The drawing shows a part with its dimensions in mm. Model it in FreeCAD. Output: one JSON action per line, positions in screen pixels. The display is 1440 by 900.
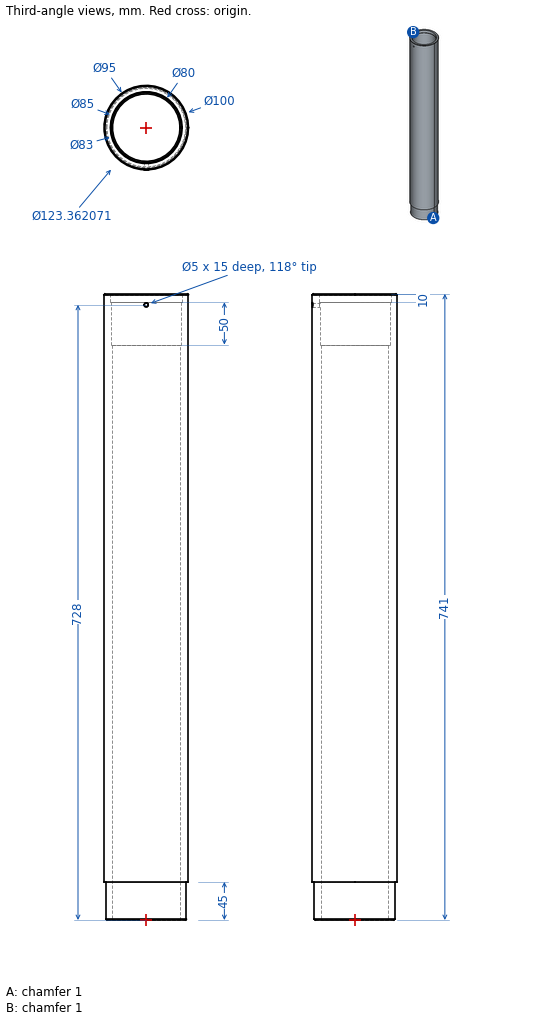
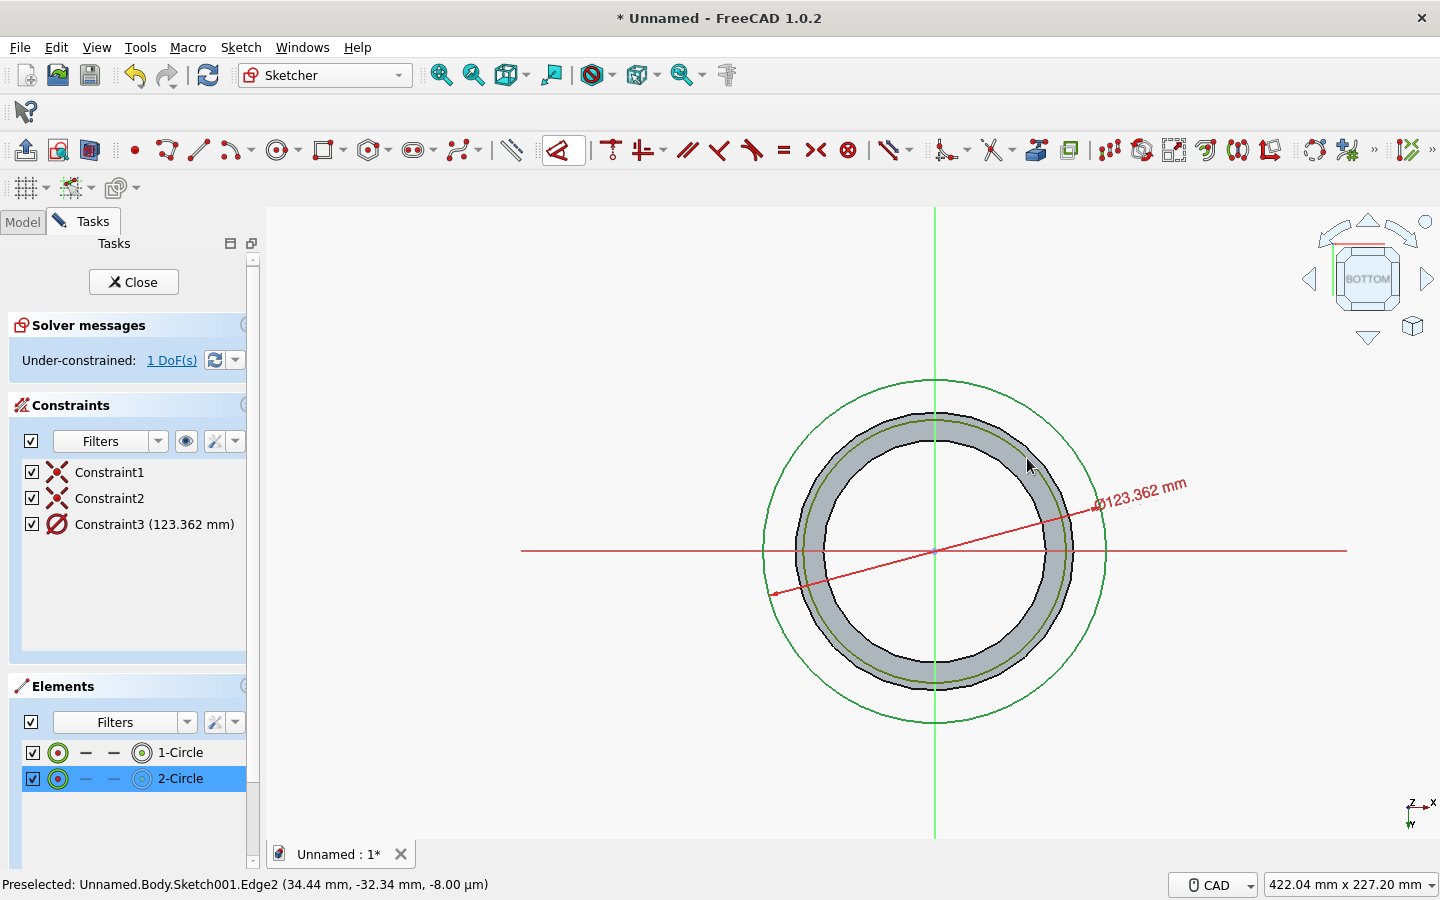
{"action": "left_click", "coordinate": [580, 150]}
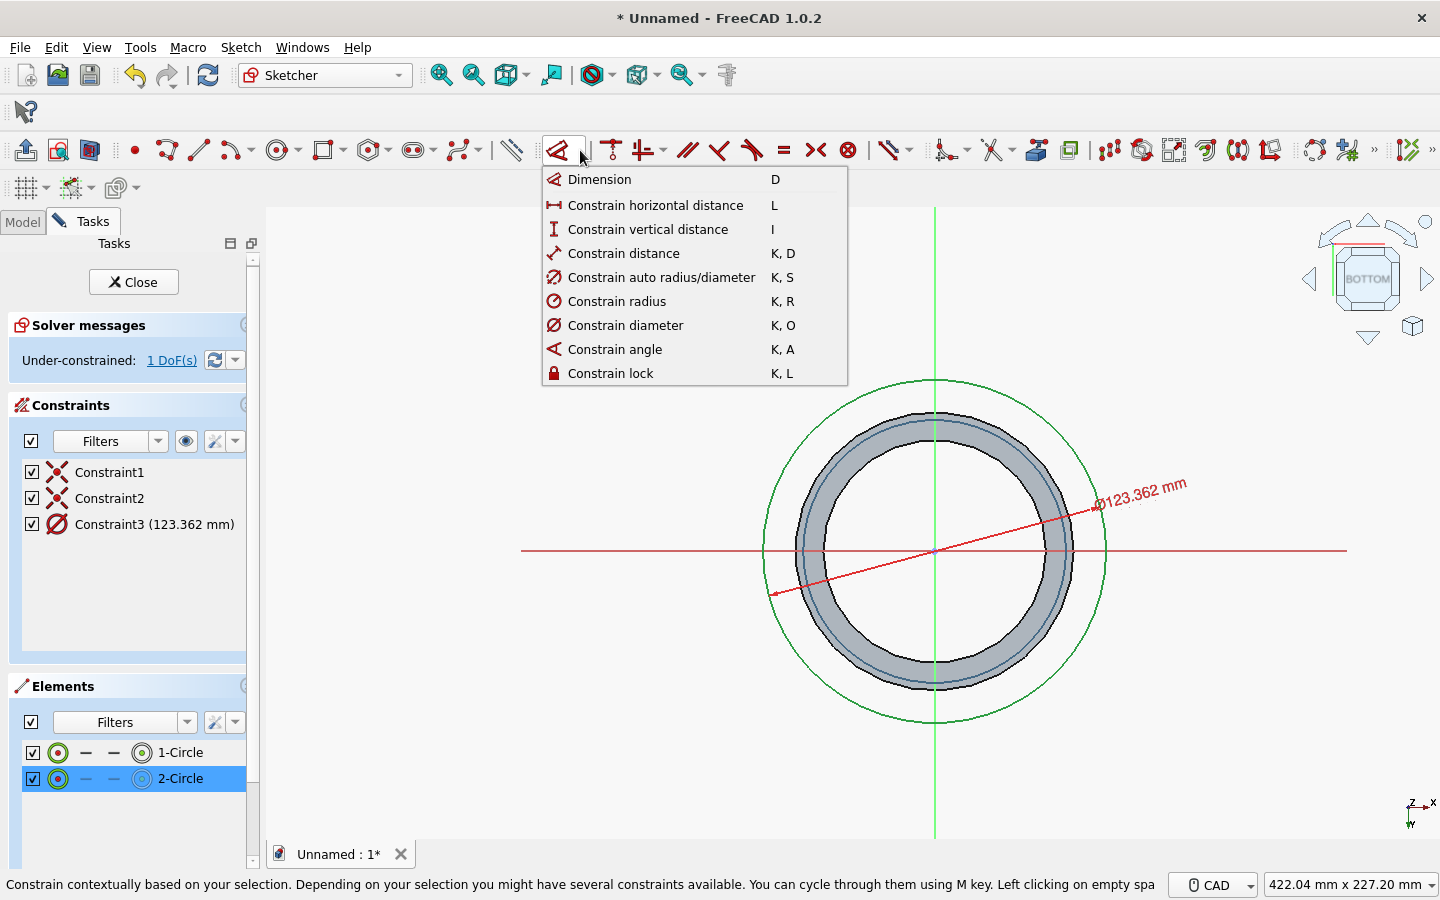
{"action": "left_click", "coordinate": [695, 325]}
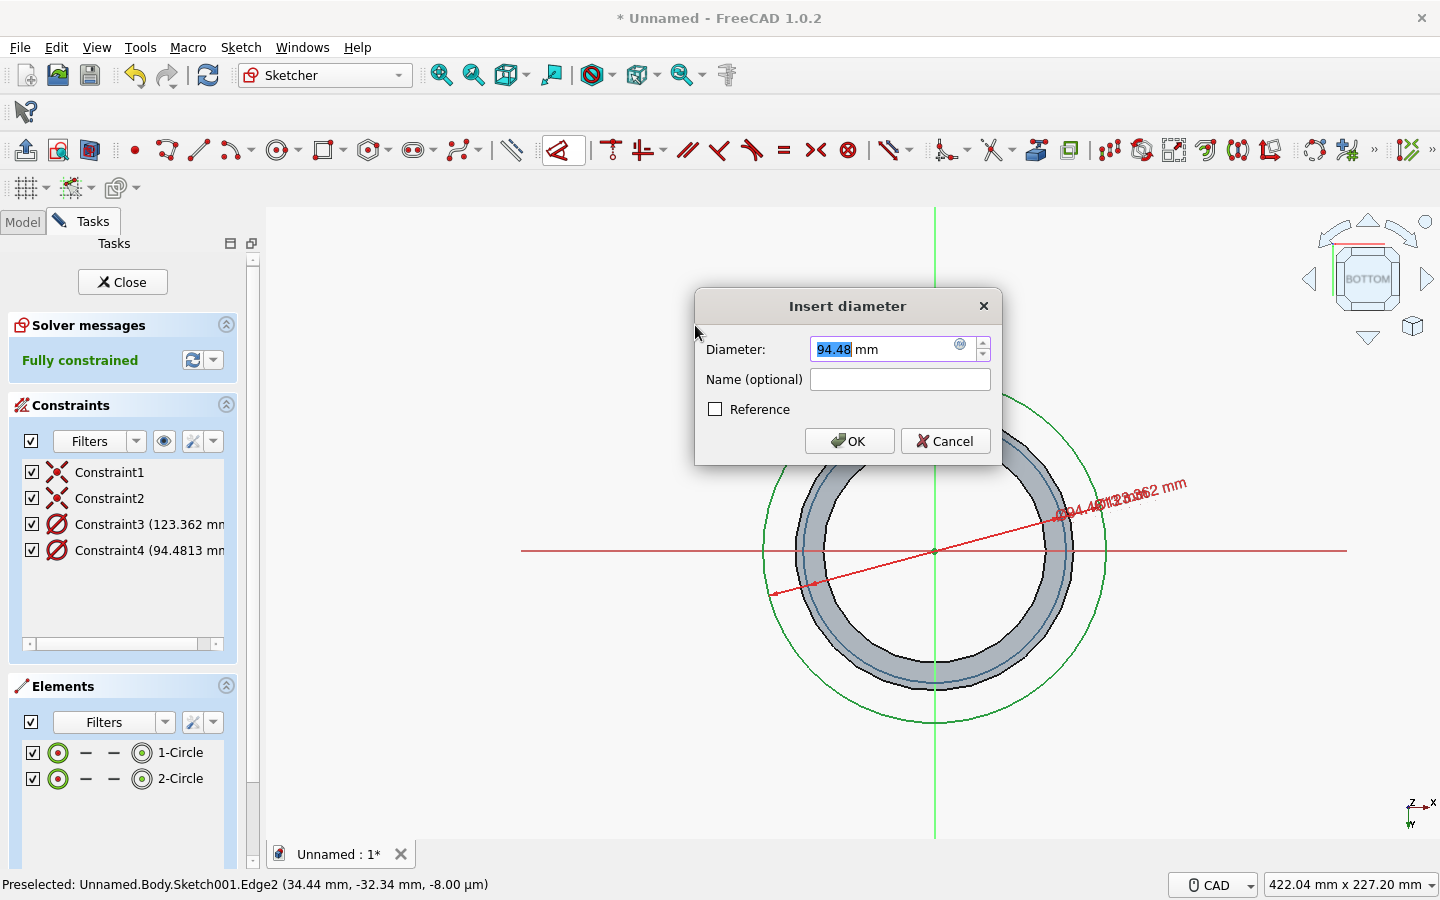
{"action": "type", "text": "95"}
{"action": "key", "text": "Return"}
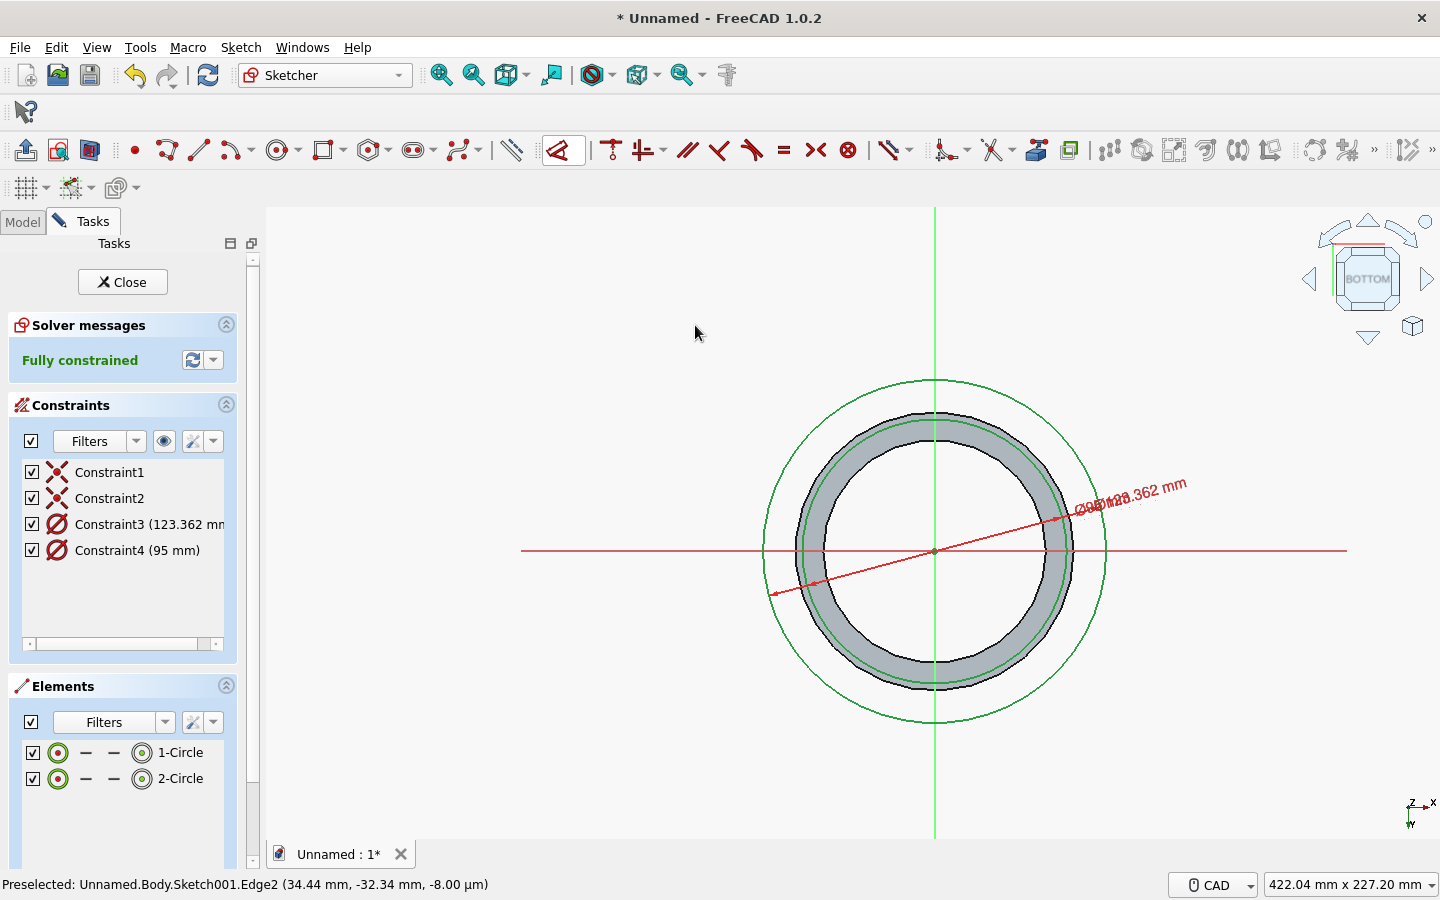
{"action": "left_click", "coordinate": [123, 282]}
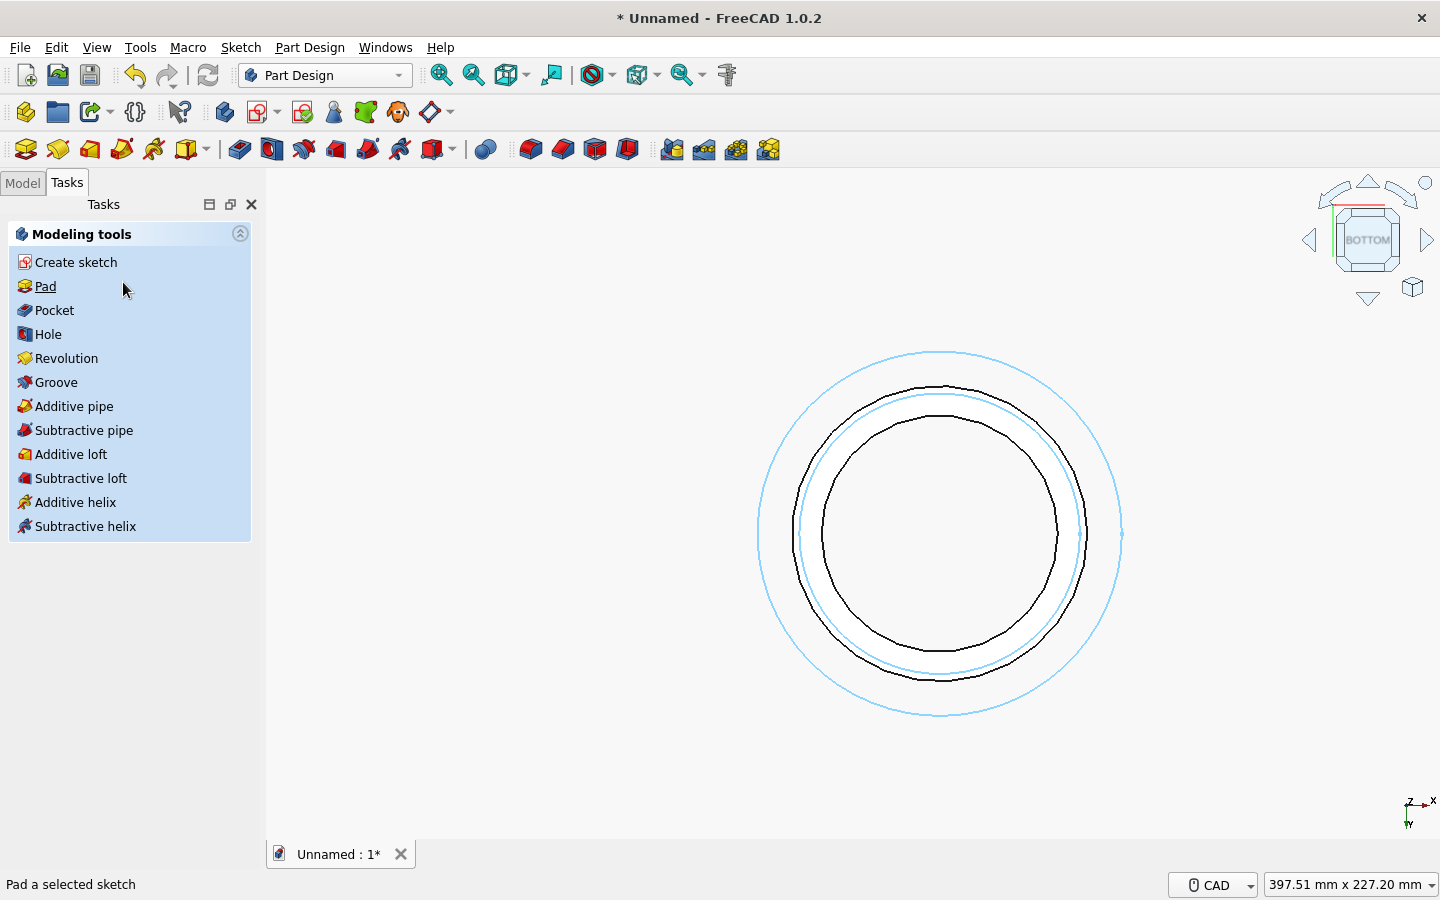
{"action": "left_click", "coordinate": [240, 150]}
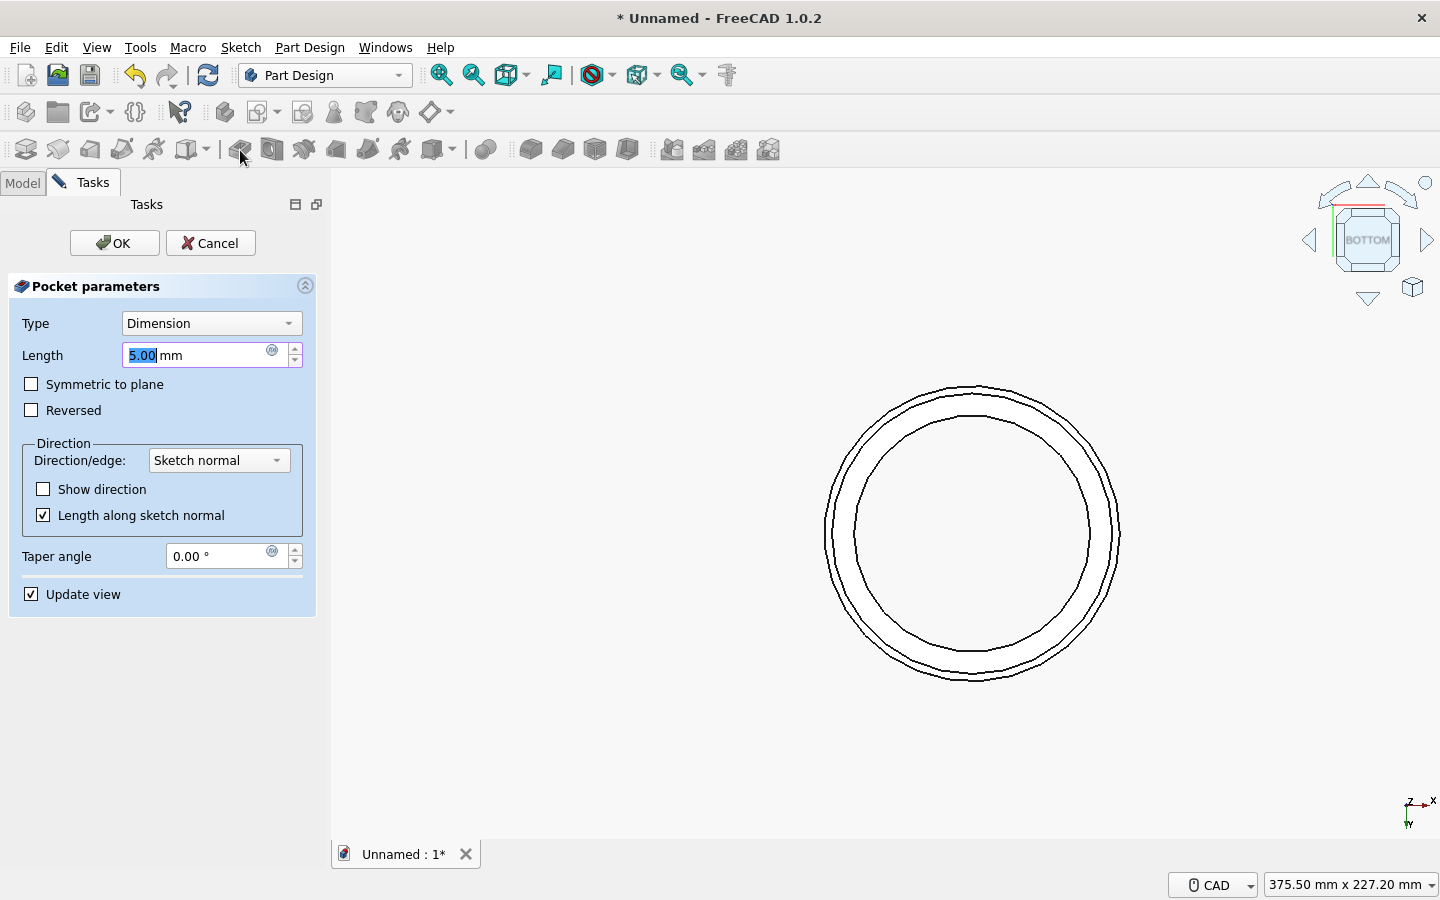
{"action": "type", "text": "45"}
{"action": "key", "text": "Tab"}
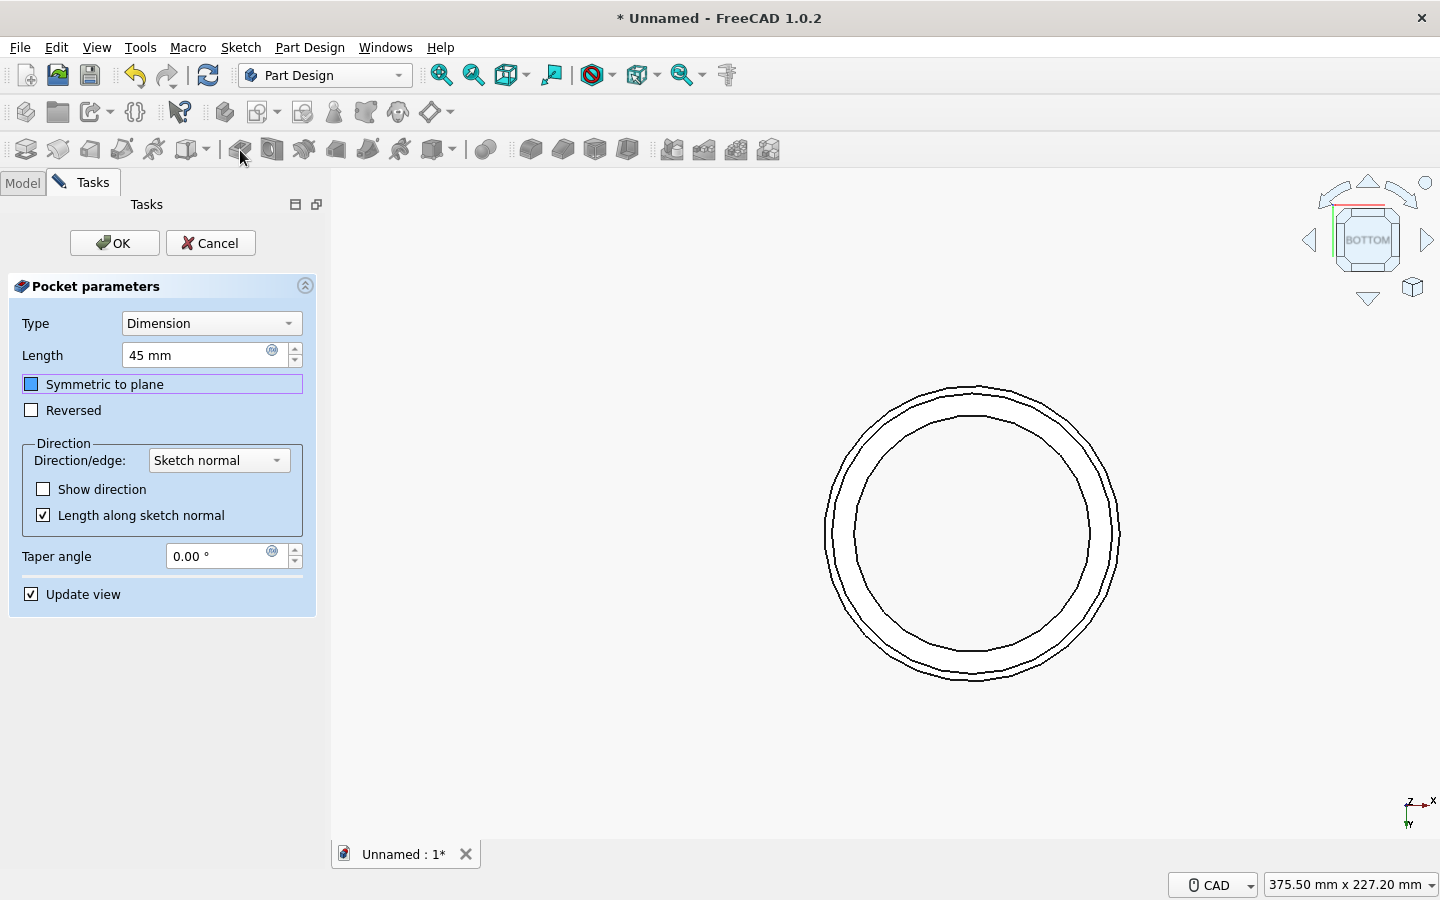
{"action": "left_click", "coordinate": [115, 243]}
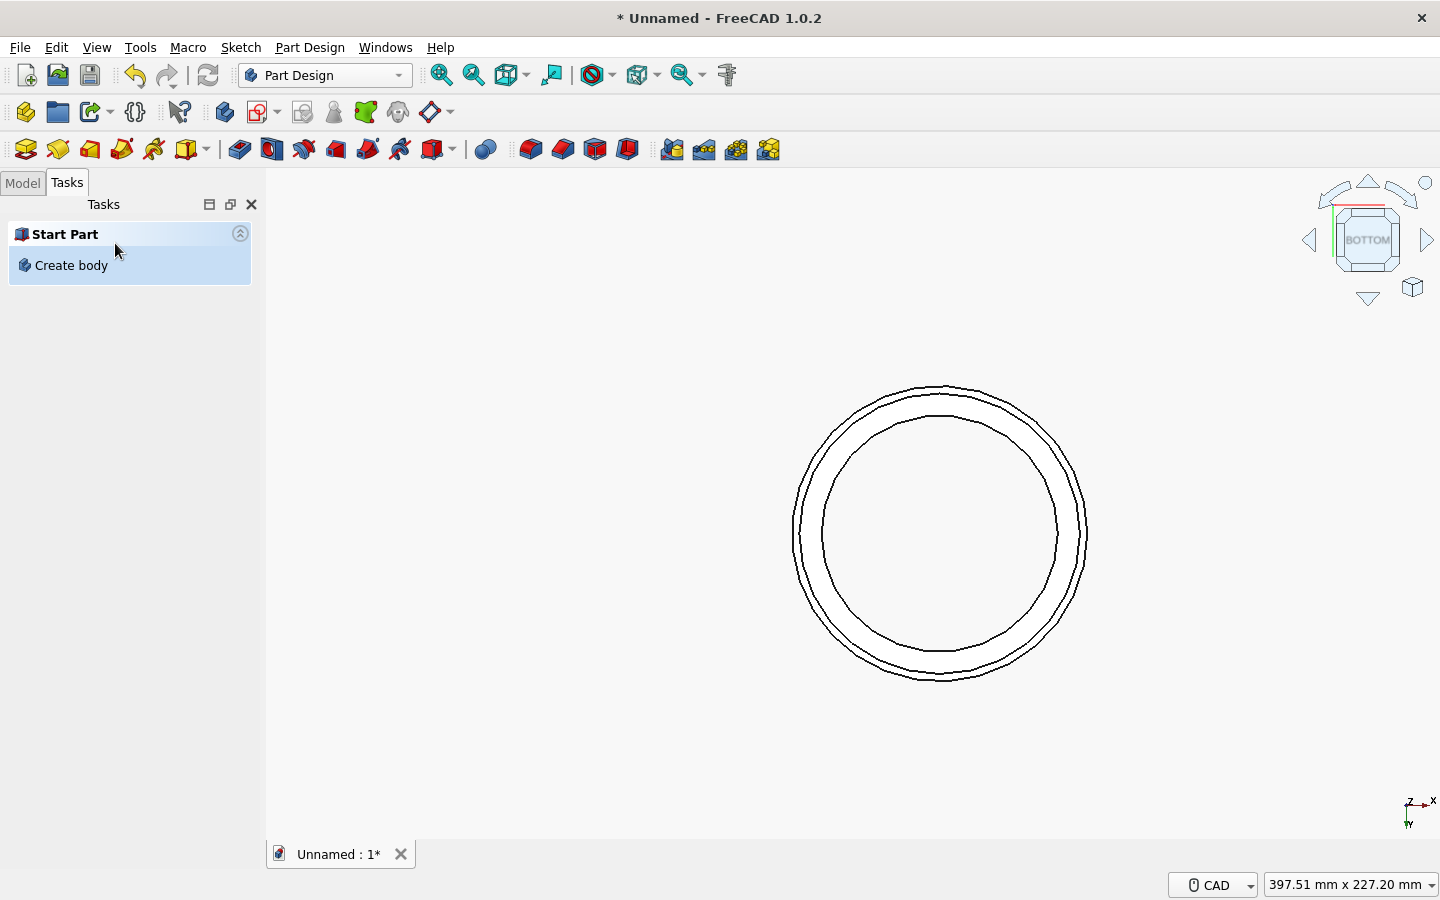
{"action": "left_click", "coordinate": [442, 76]}